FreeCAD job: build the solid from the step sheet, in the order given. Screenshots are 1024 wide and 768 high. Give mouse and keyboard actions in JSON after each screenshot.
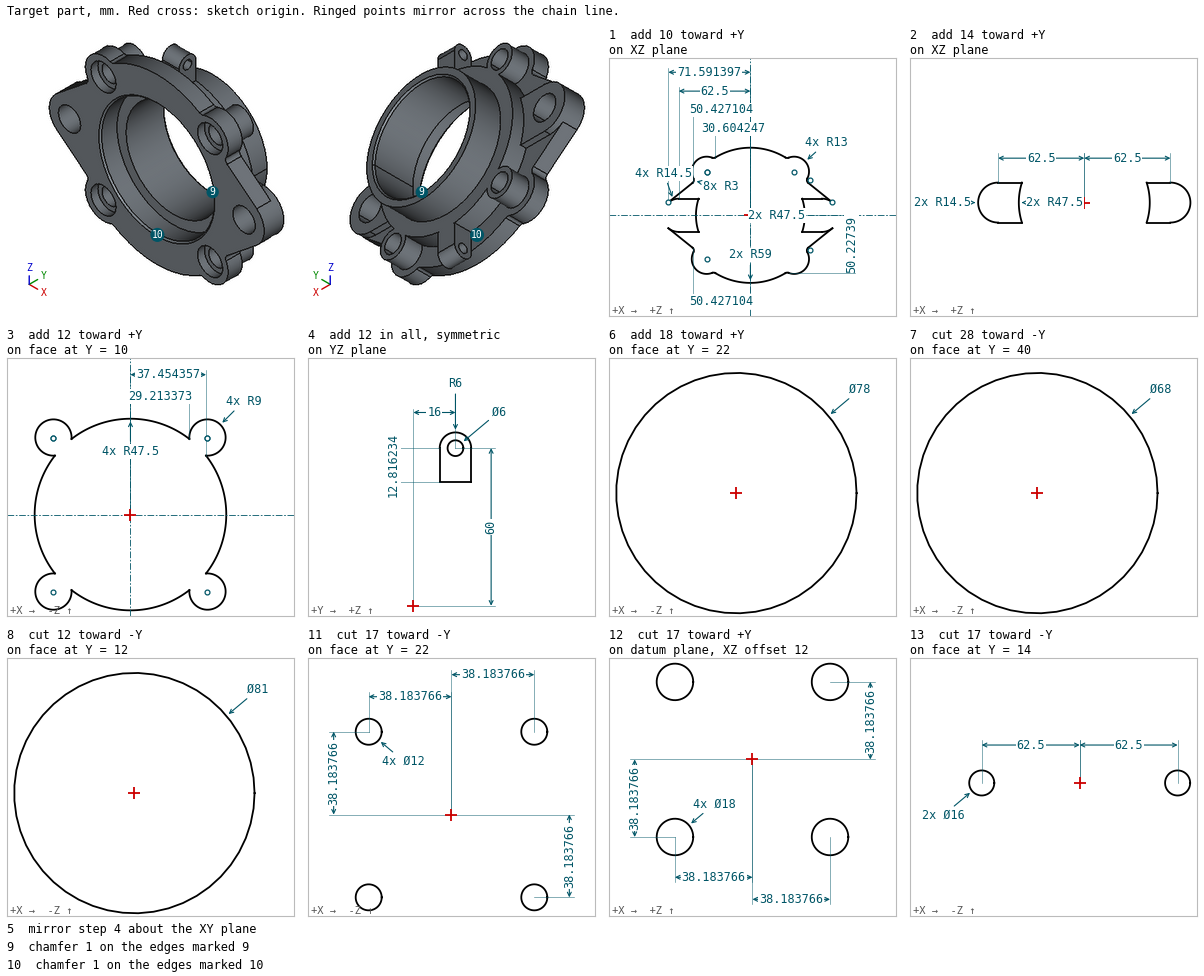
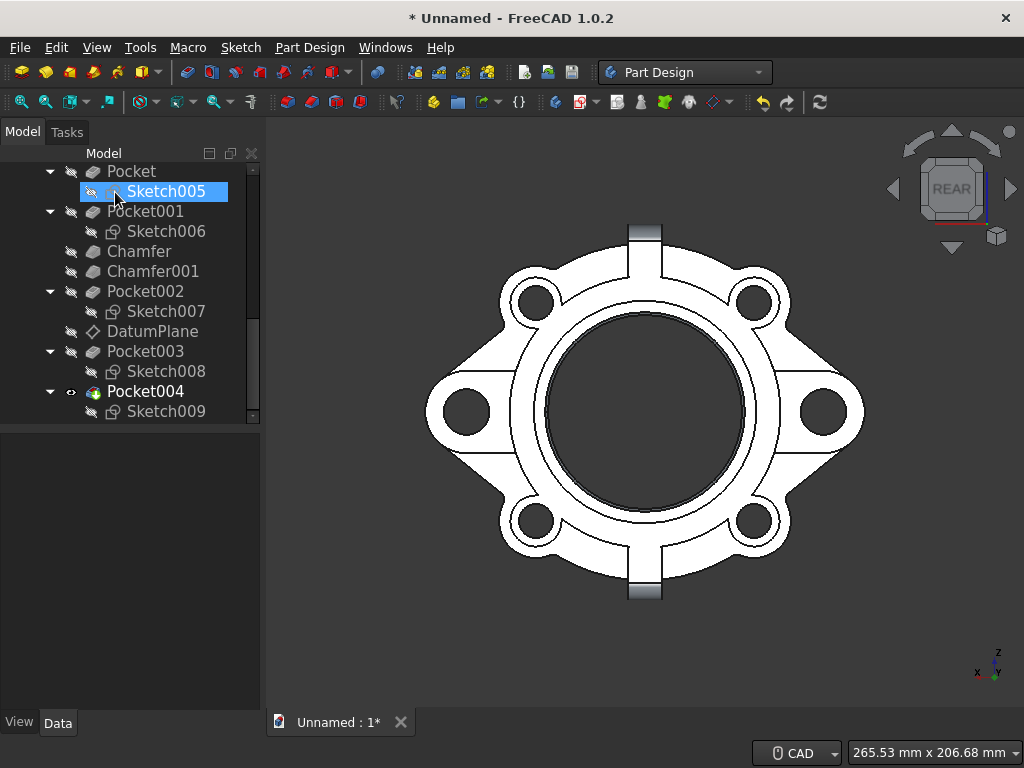
{"action": "key", "text": "0"}